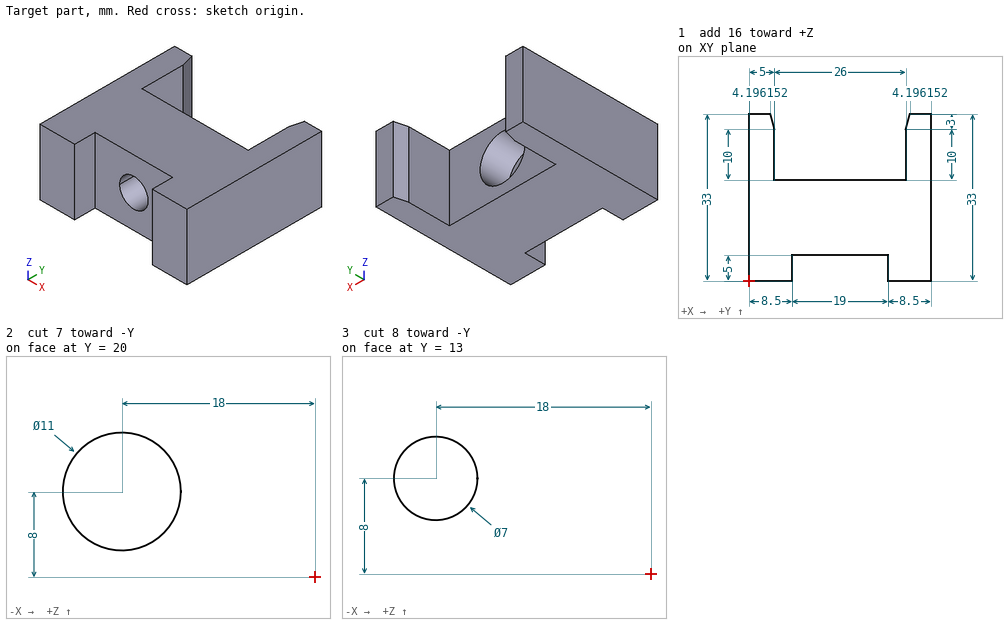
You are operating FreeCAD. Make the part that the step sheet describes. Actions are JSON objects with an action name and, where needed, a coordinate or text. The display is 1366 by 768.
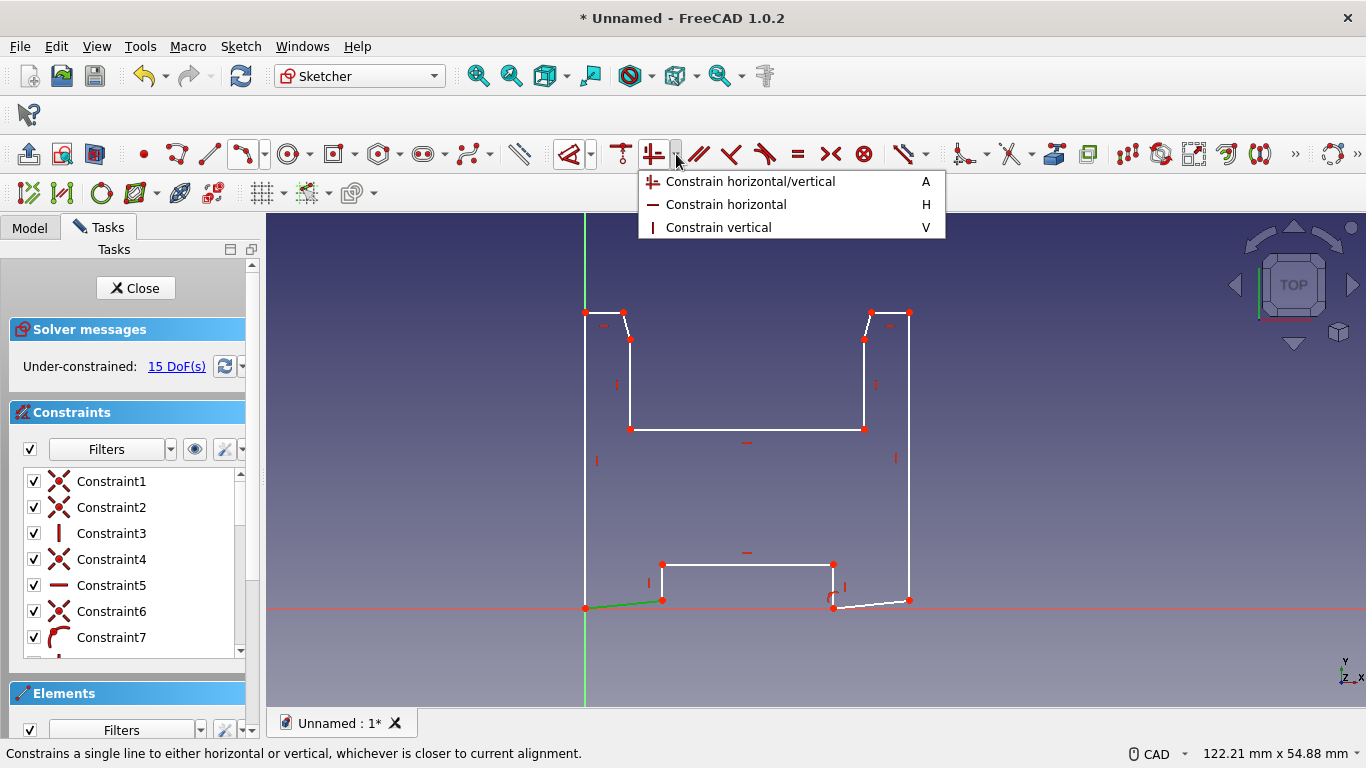
{"action": "left_click", "coordinate": [792, 204]}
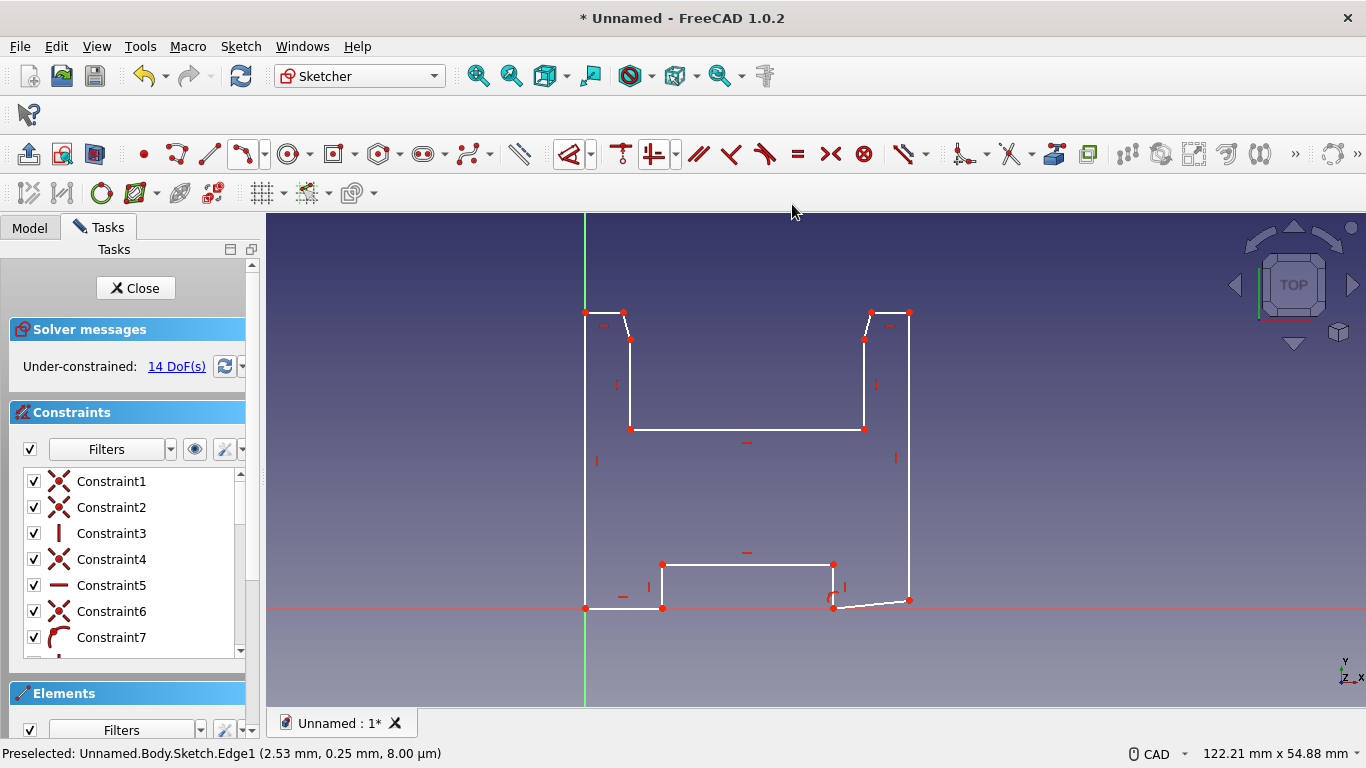
{"action": "left_click", "coordinate": [856, 606]}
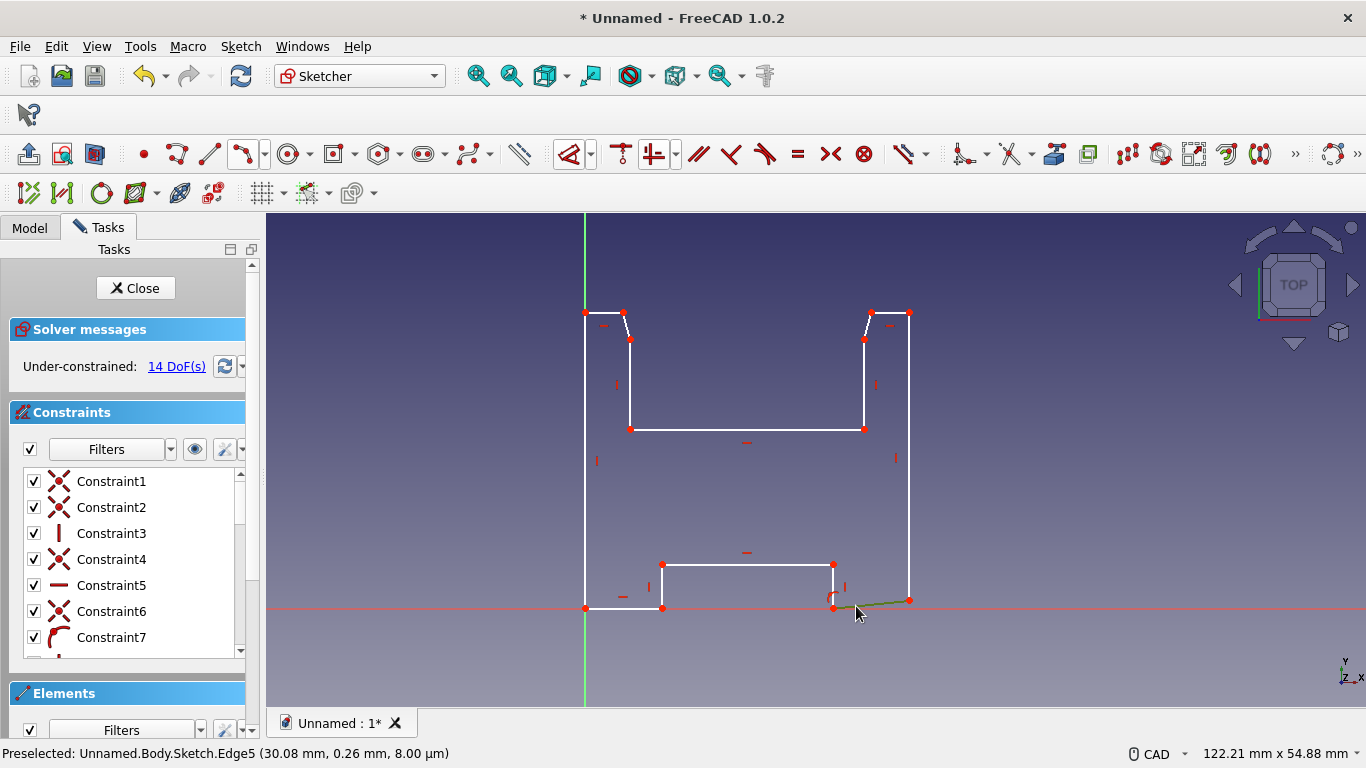
{"action": "key", "text": "h"}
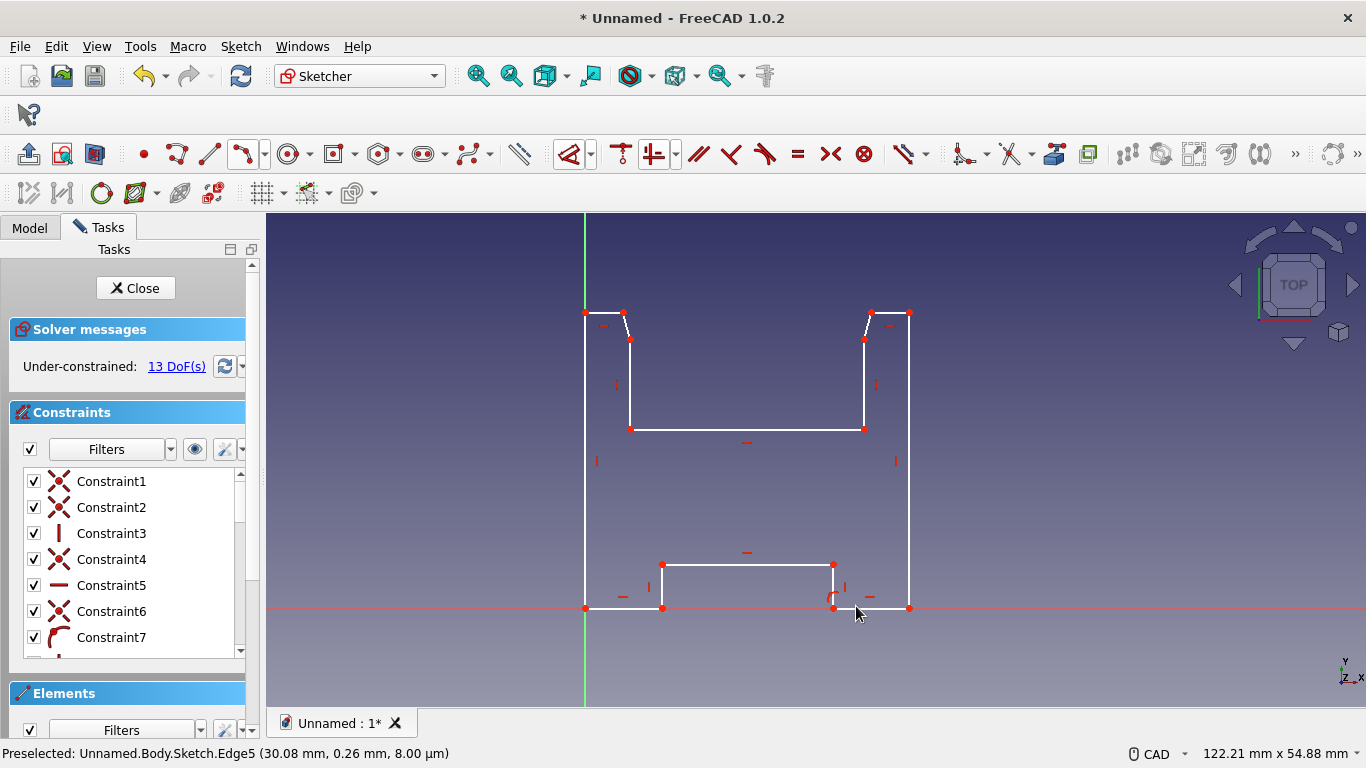
{"action": "left_click", "coordinate": [568, 154]}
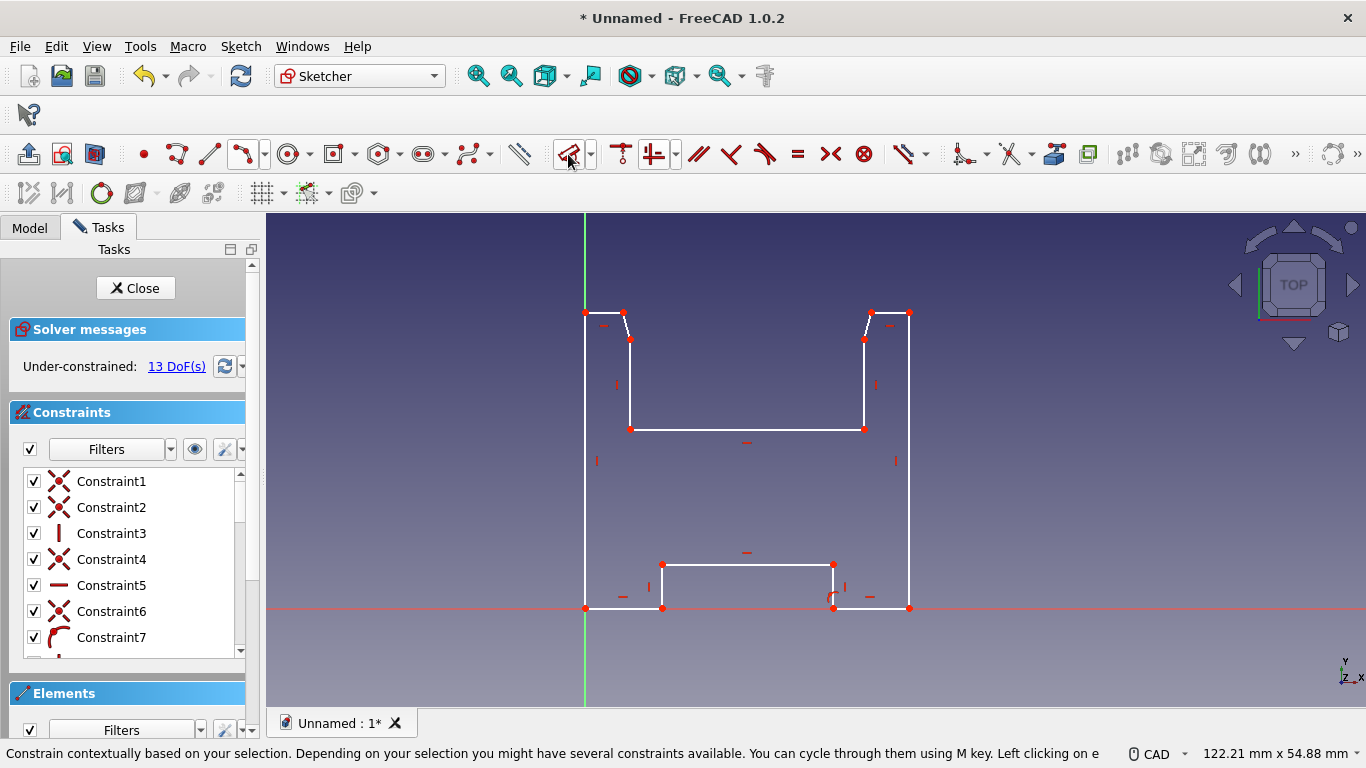
{"action": "left_click", "coordinate": [662, 596]}
{"action": "left_click", "coordinate": [628, 587]}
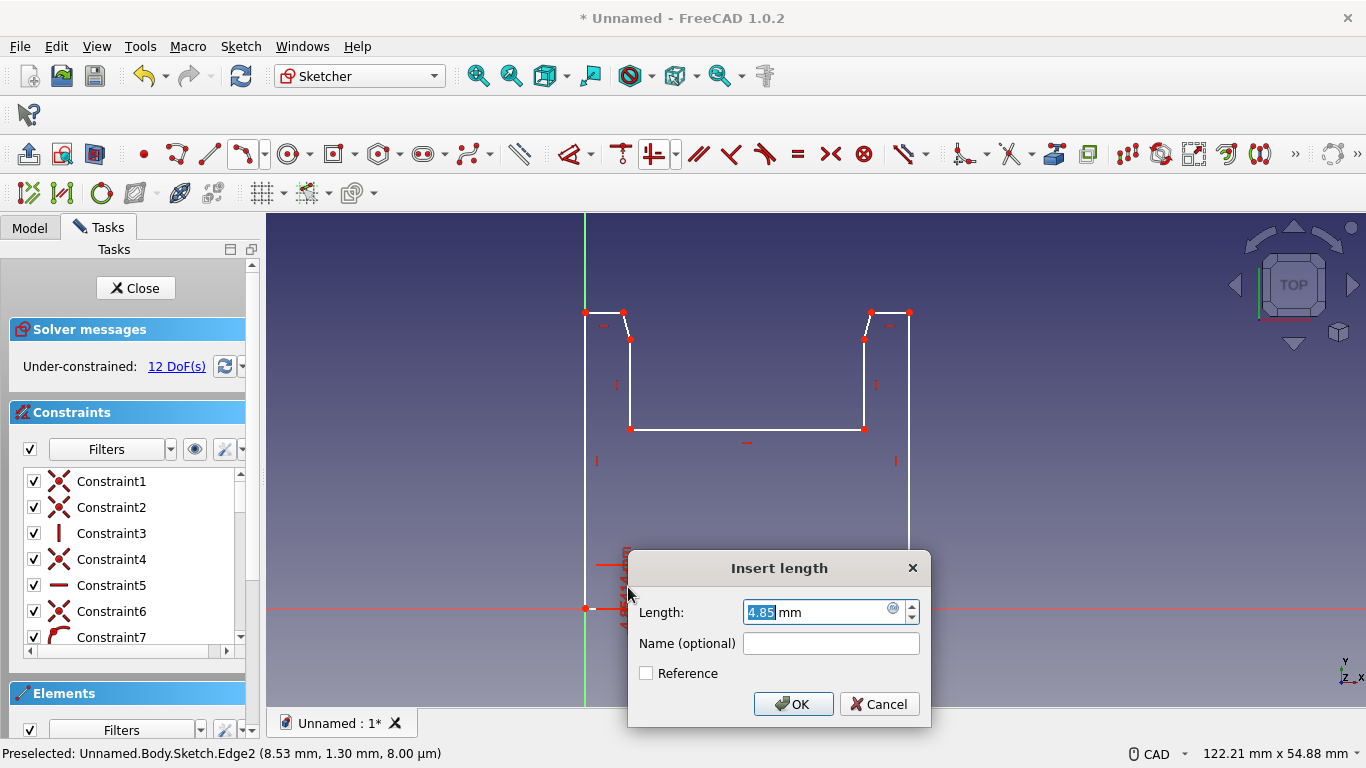
{"action": "type", "text": "5"}
{"action": "key", "text": "Return"}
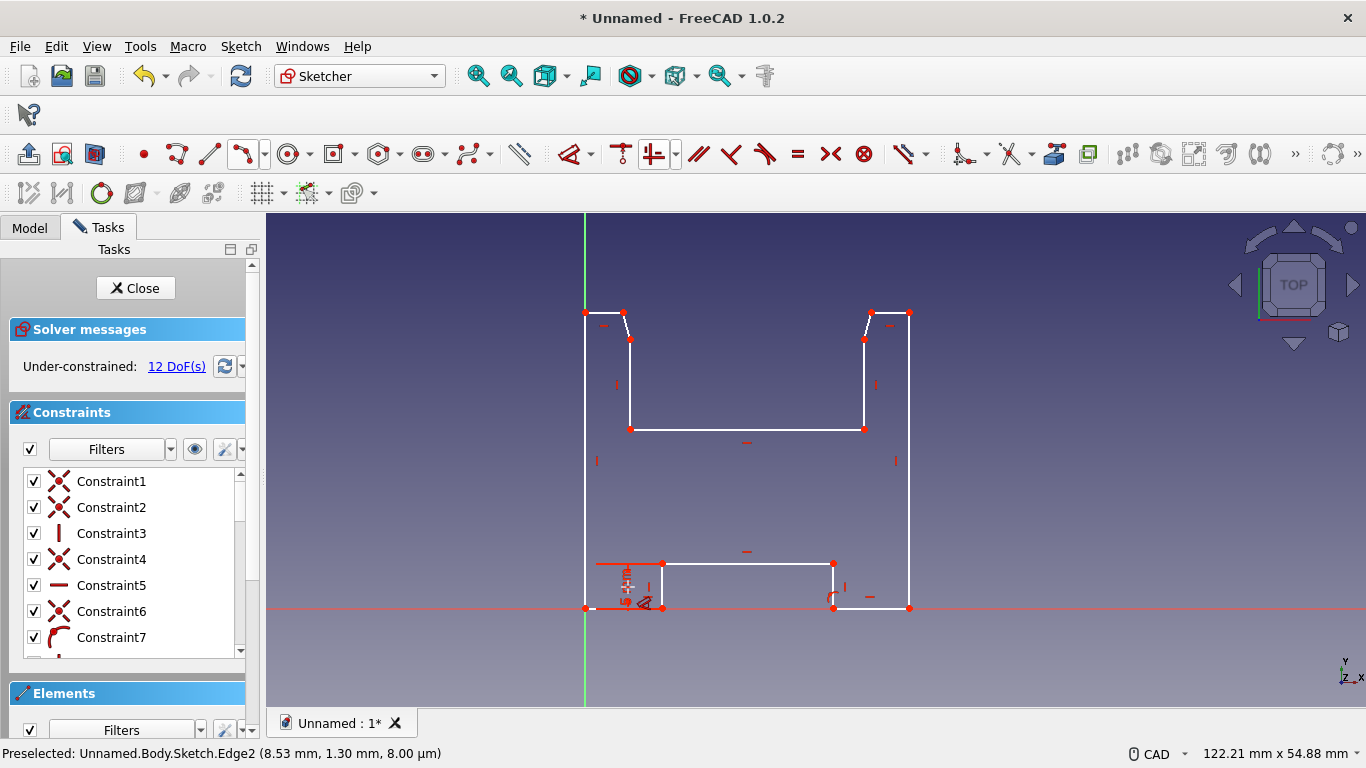
{"action": "left_click", "coordinate": [713, 564]}
{"action": "left_click", "coordinate": [747, 530]}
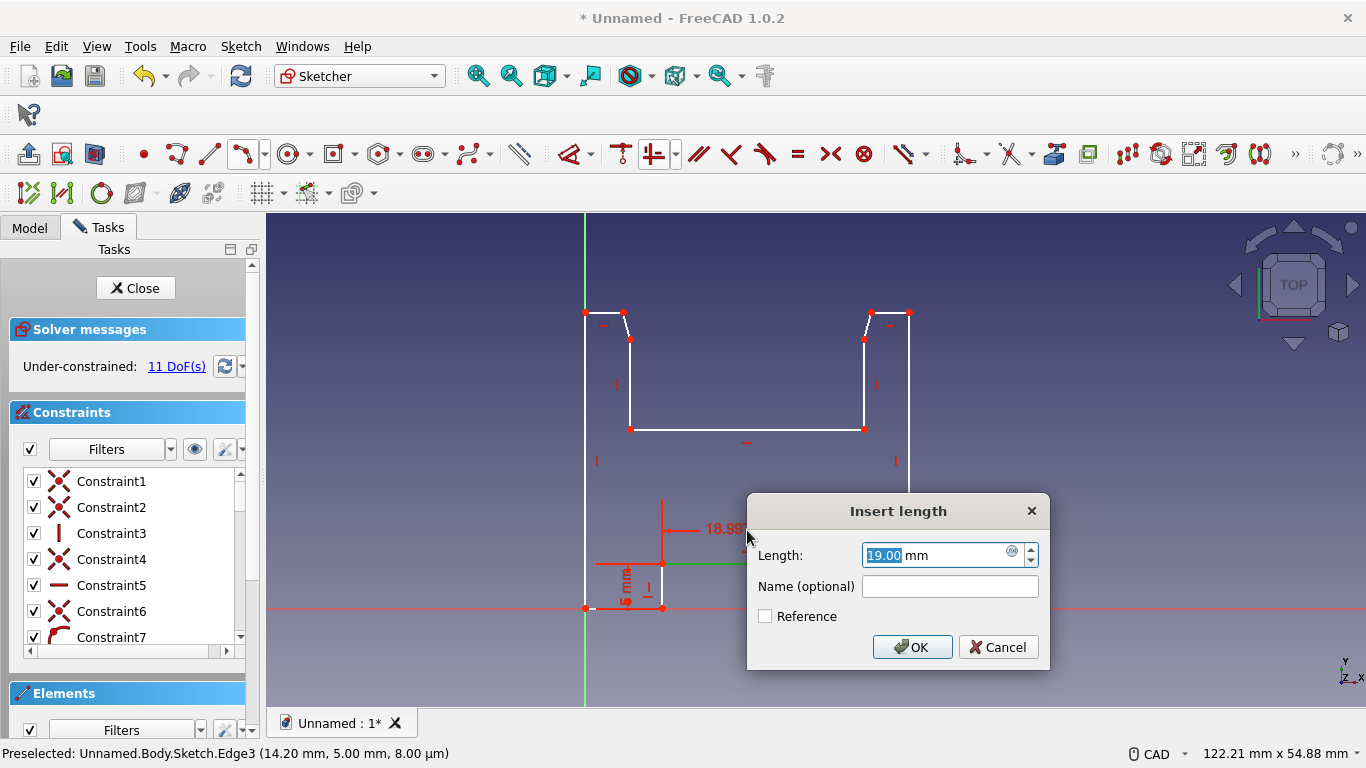
{"action": "type", "text": "19"}
{"action": "key", "text": "Return"}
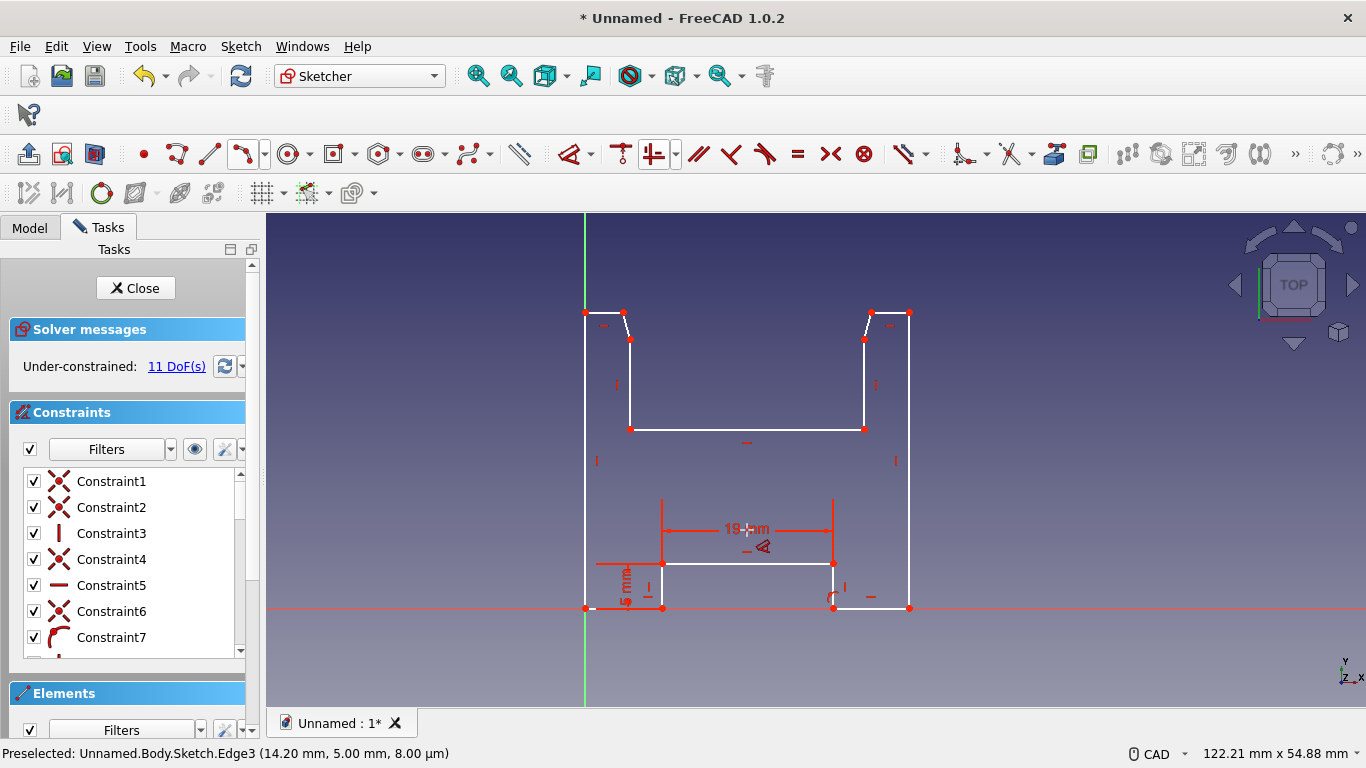
{"action": "left_click", "coordinate": [909, 520]}
{"action": "left_click", "coordinate": [943, 461]}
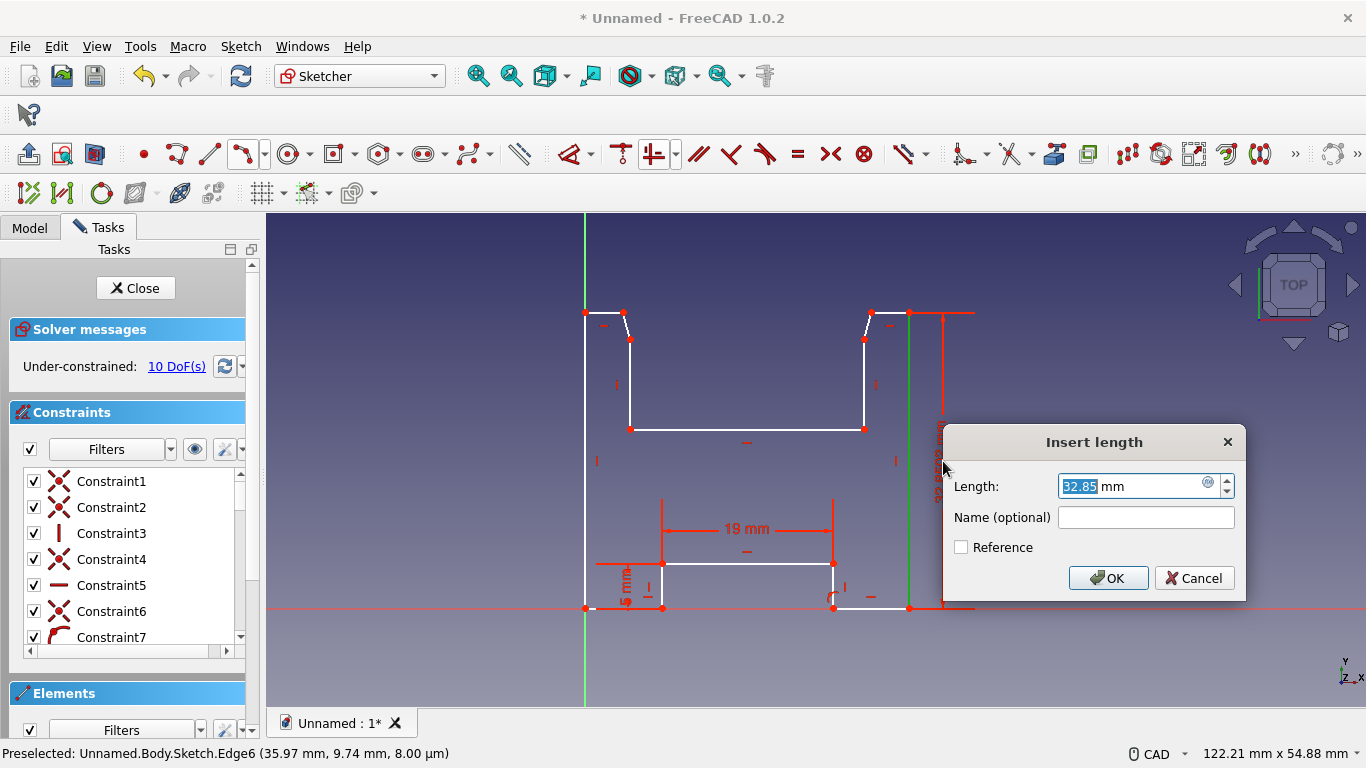
{"action": "type", "text": "33"}
{"action": "key", "text": "Return"}